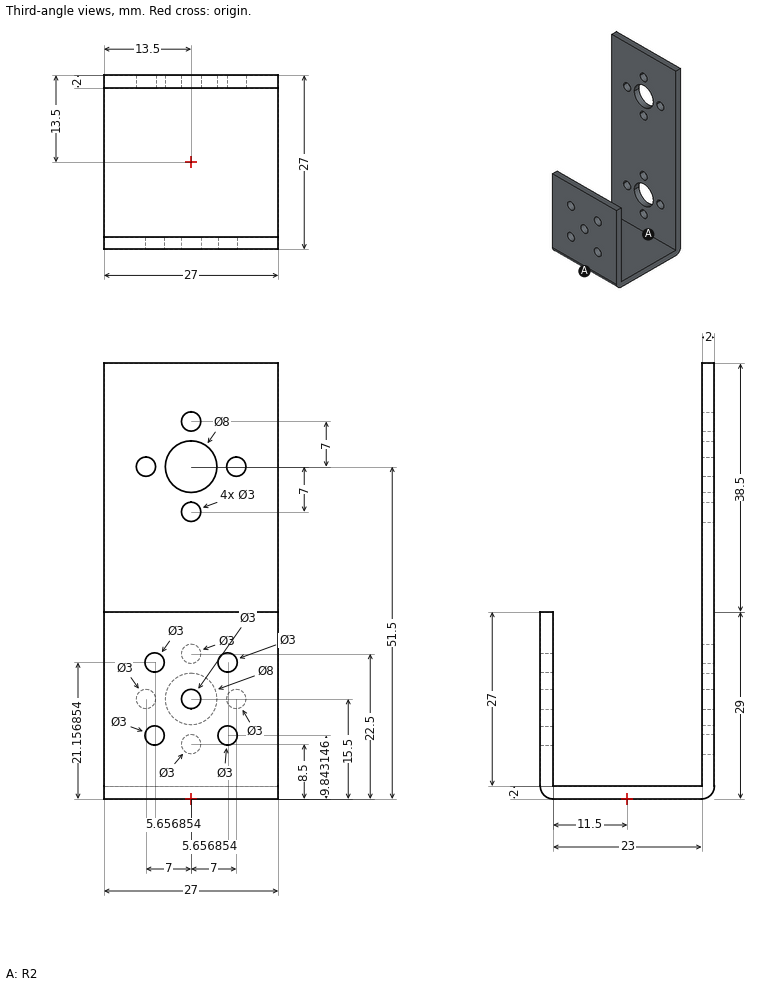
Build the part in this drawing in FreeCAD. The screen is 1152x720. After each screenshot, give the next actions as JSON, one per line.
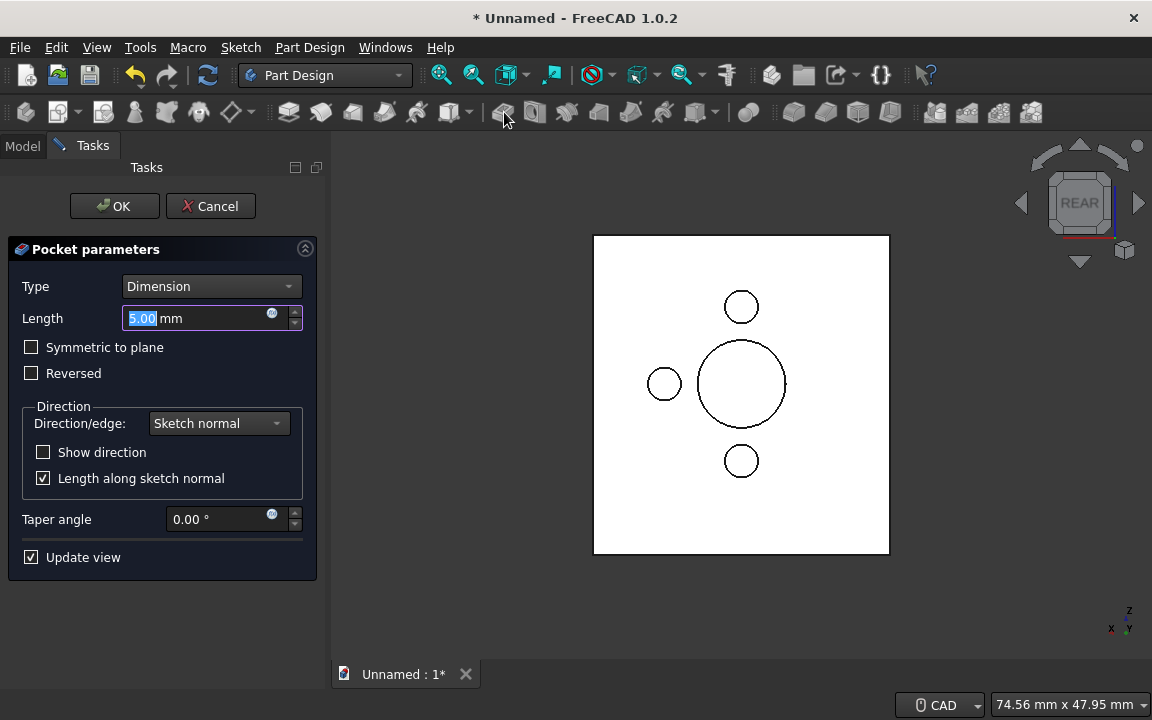
{"action": "left_click", "coordinate": [212, 286]}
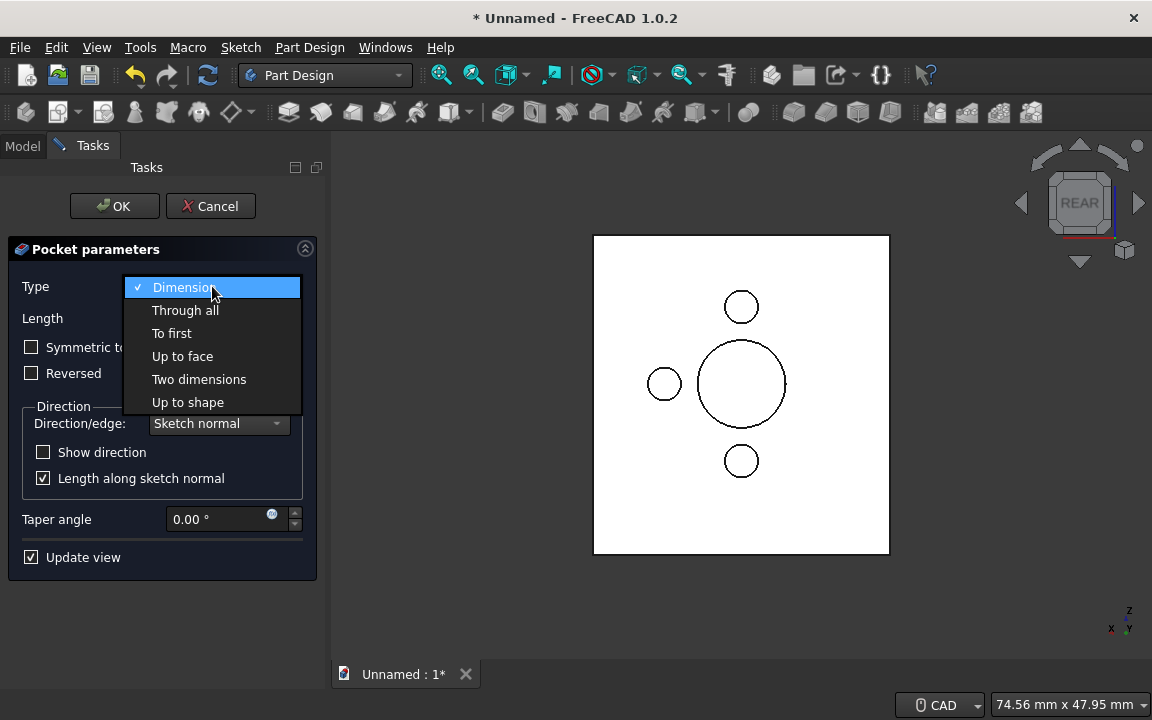
{"action": "left_click", "coordinate": [212, 334]}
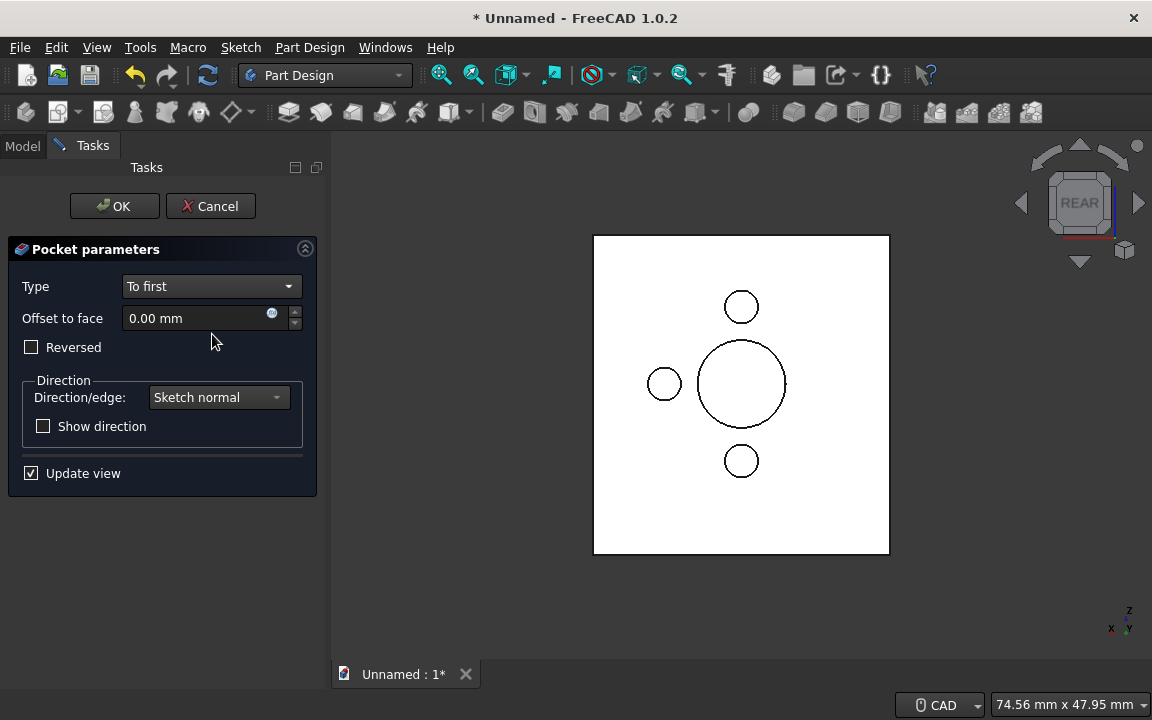
{"action": "left_click", "coordinate": [115, 206]}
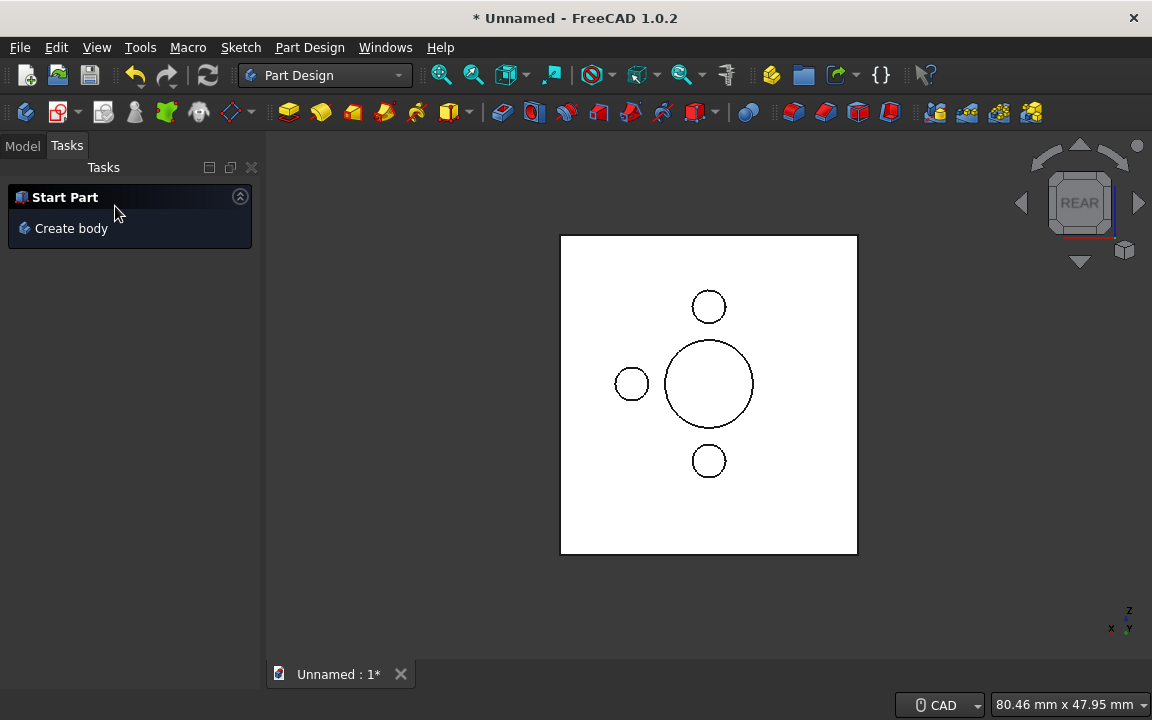
{"action": "left_click", "coordinate": [624, 303]}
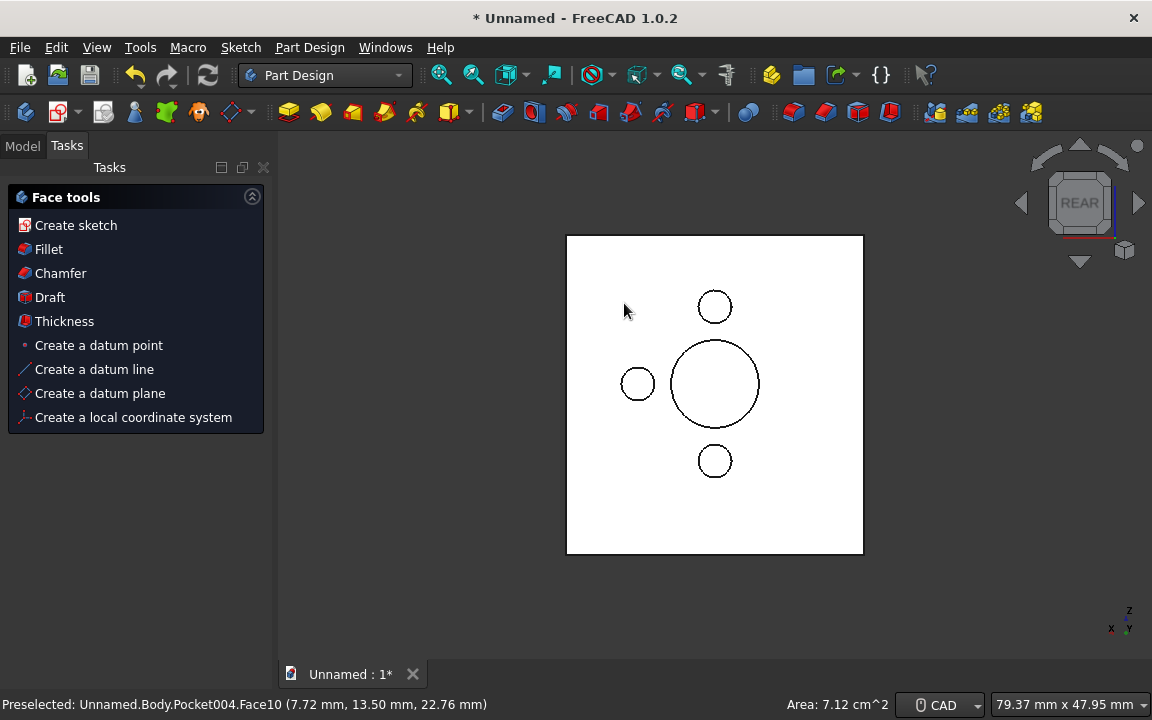
{"action": "left_click", "coordinate": [58, 112]}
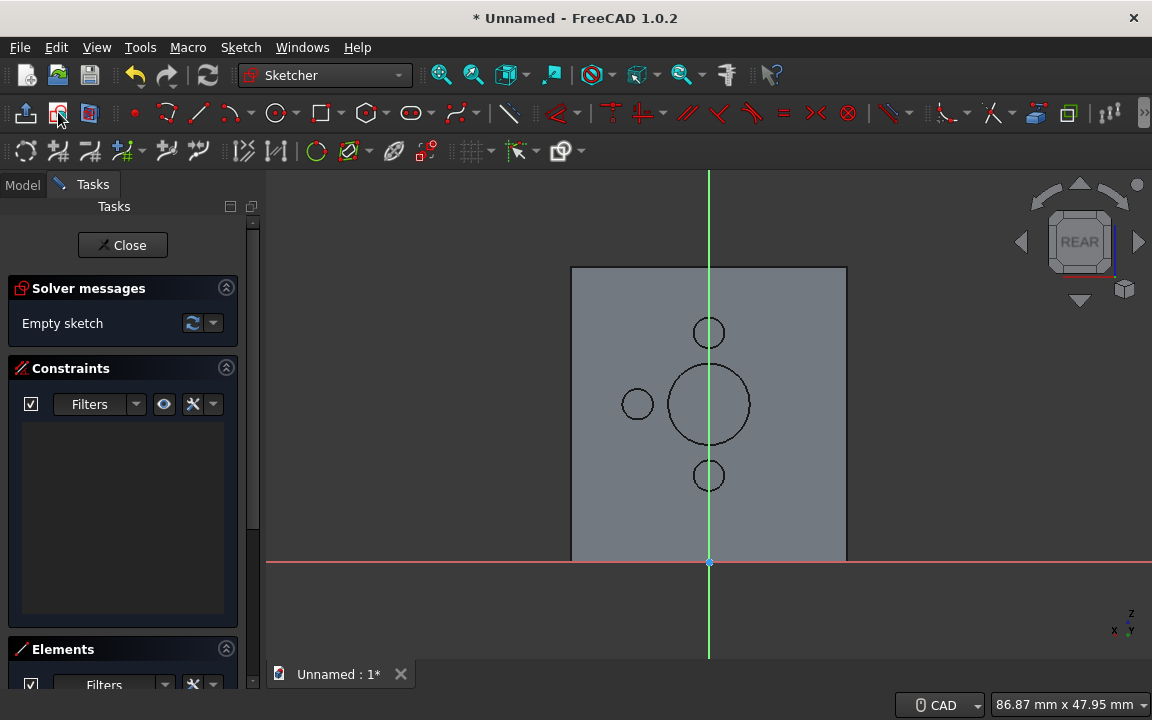
{"action": "scroll", "coordinate": [794, 403], "scroll_direction": "up", "scroll_amount": 12}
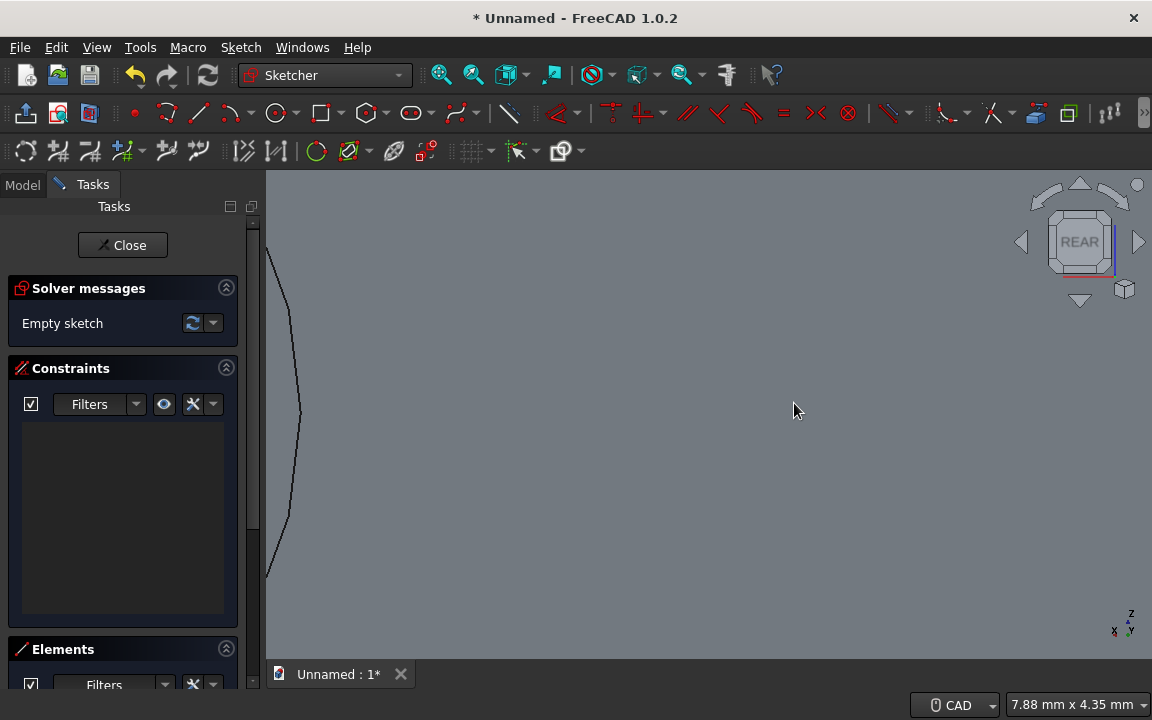
{"action": "key", "text": "g c"}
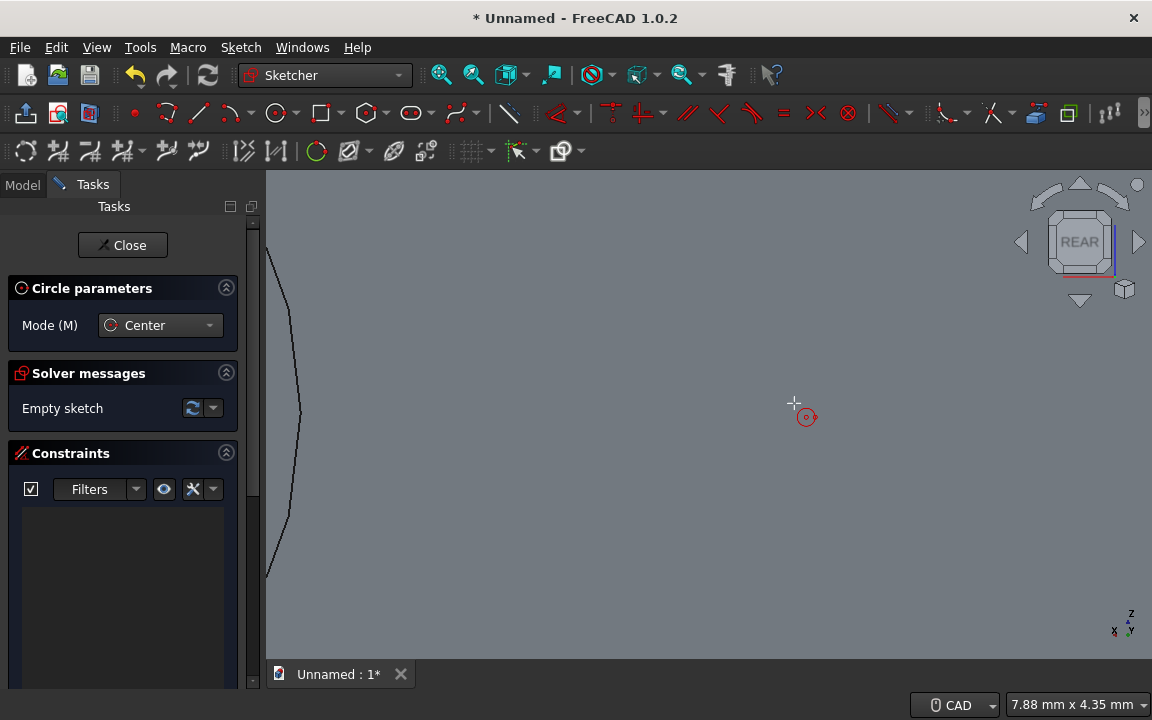
{"action": "left_click", "coordinate": [638, 413]}
{"action": "left_click", "coordinate": [757, 293]}
{"action": "key", "text": "Escape"}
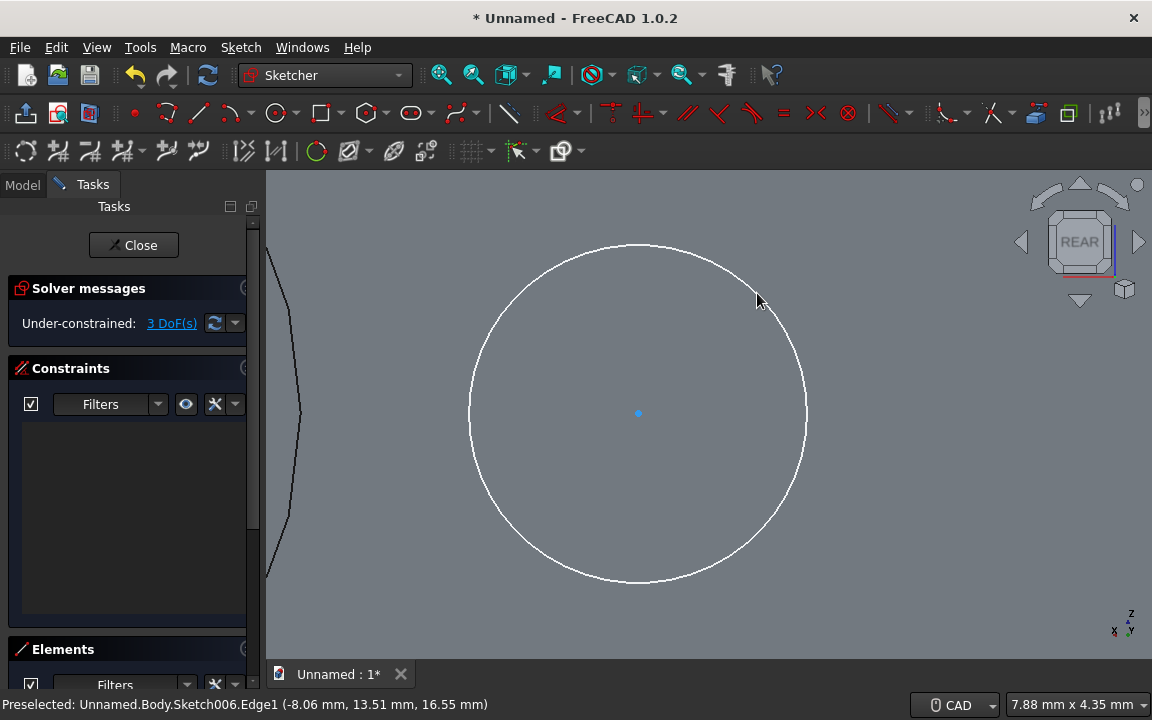
{"action": "key", "text": "d"}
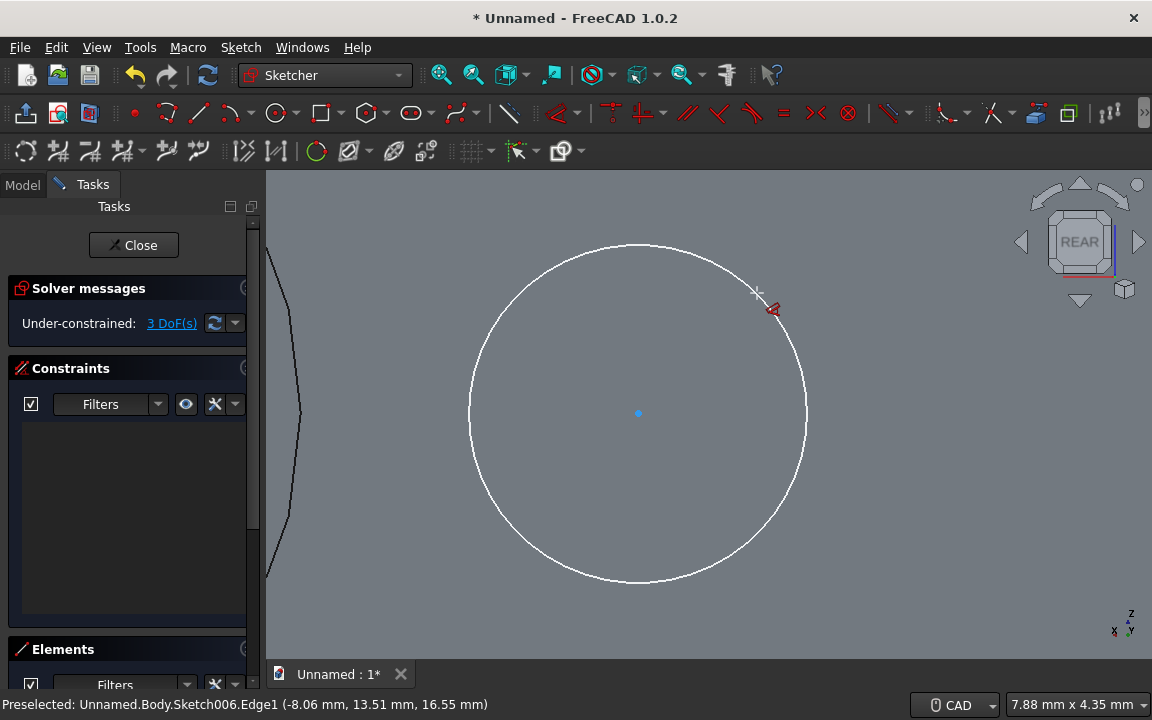
{"action": "left_click", "coordinate": [757, 294]}
{"action": "left_click", "coordinate": [780, 271]}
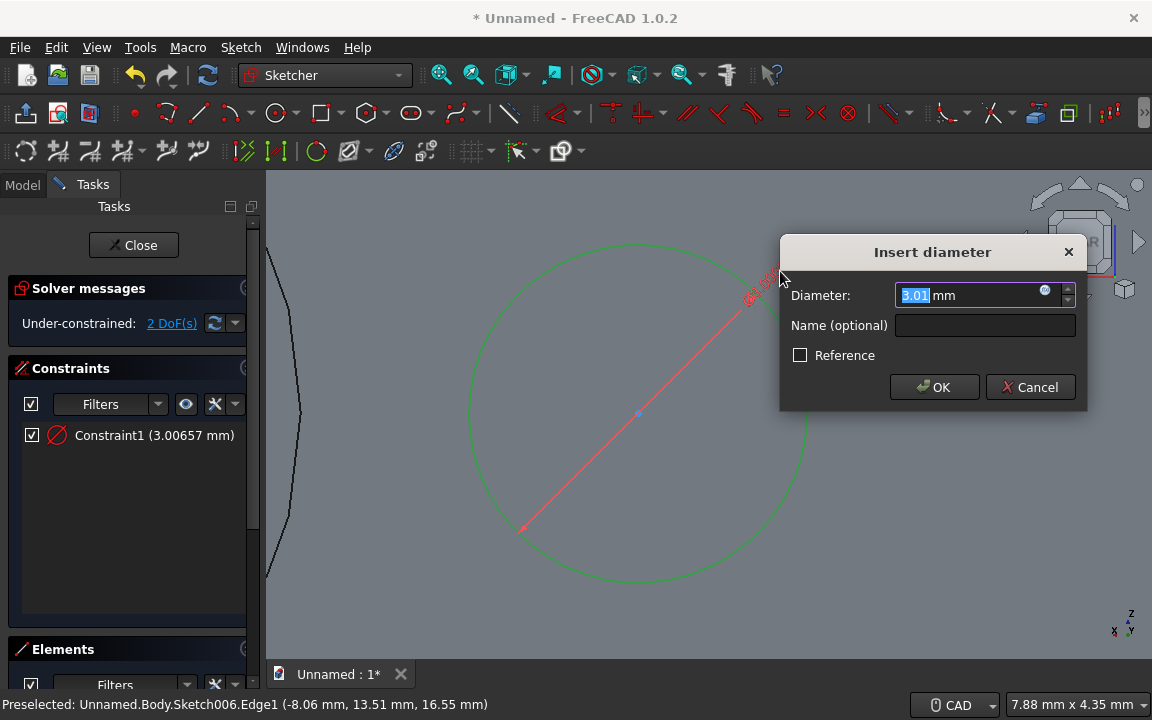
{"action": "type", "text": "3"}
{"action": "key", "text": "Return"}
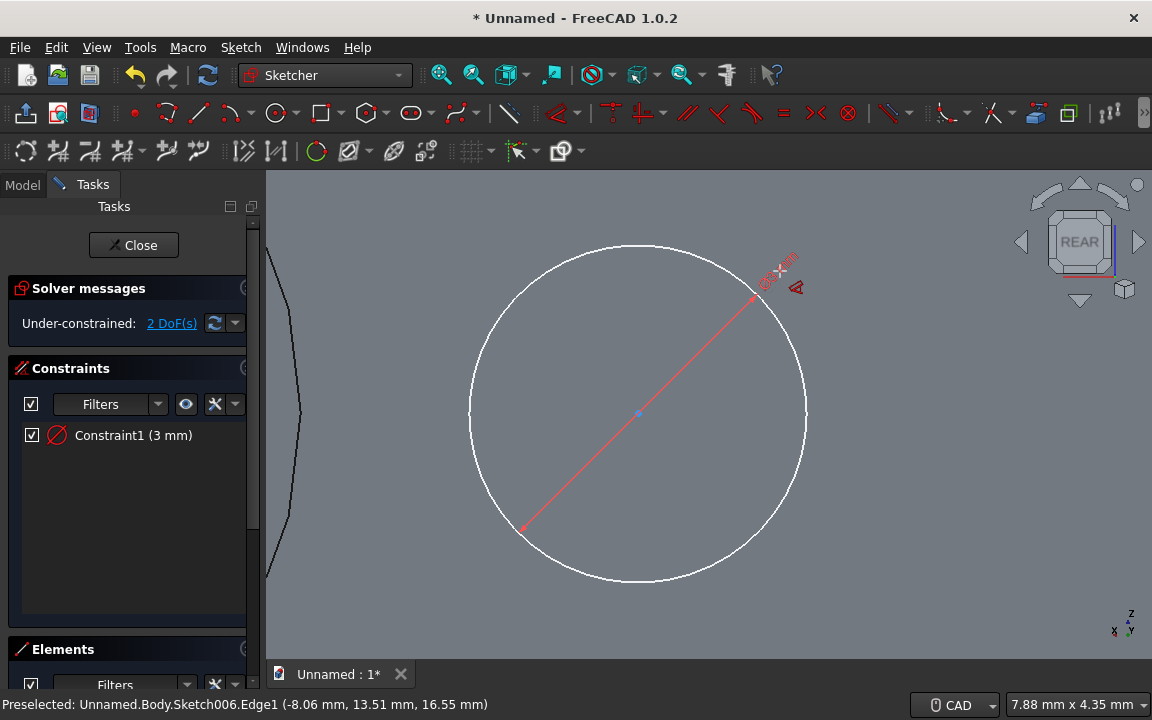
{"action": "left_click", "coordinate": [638, 414]}
{"action": "left_click", "coordinate": [387, 380]}